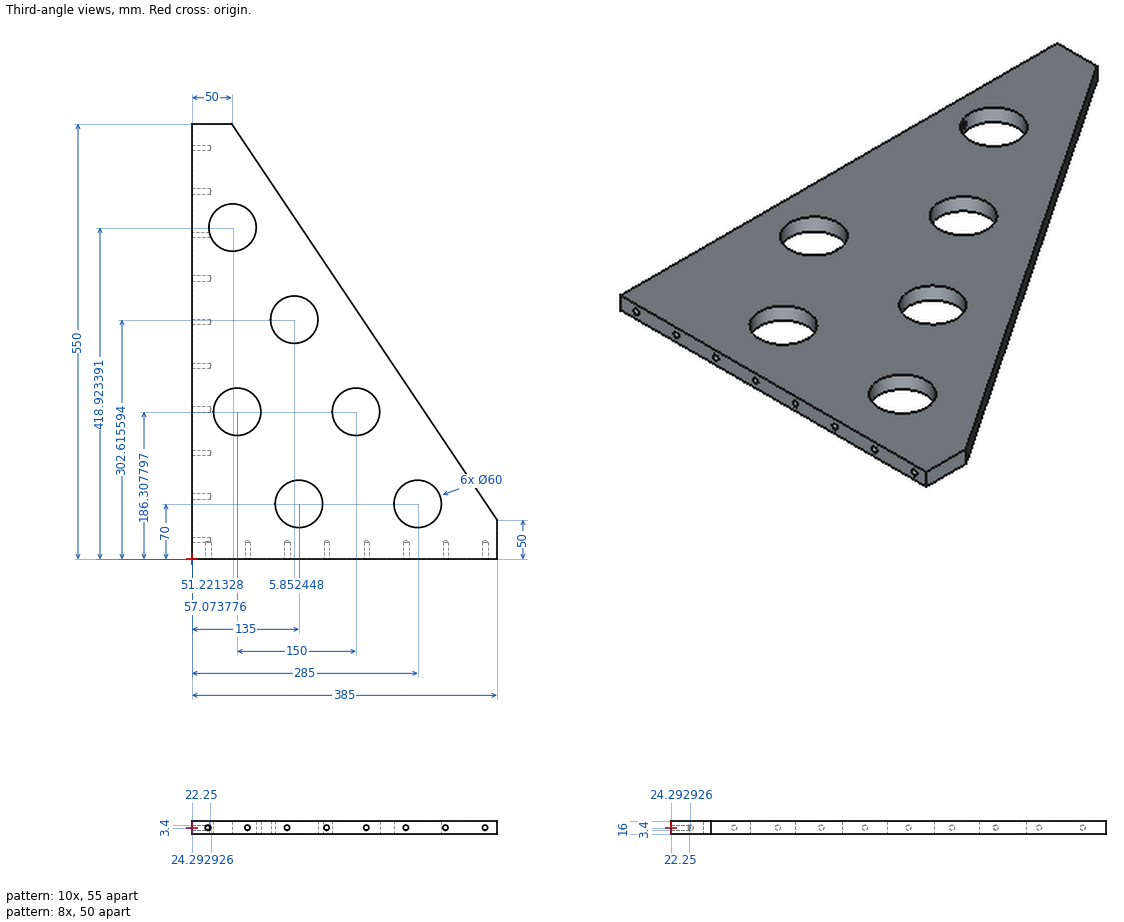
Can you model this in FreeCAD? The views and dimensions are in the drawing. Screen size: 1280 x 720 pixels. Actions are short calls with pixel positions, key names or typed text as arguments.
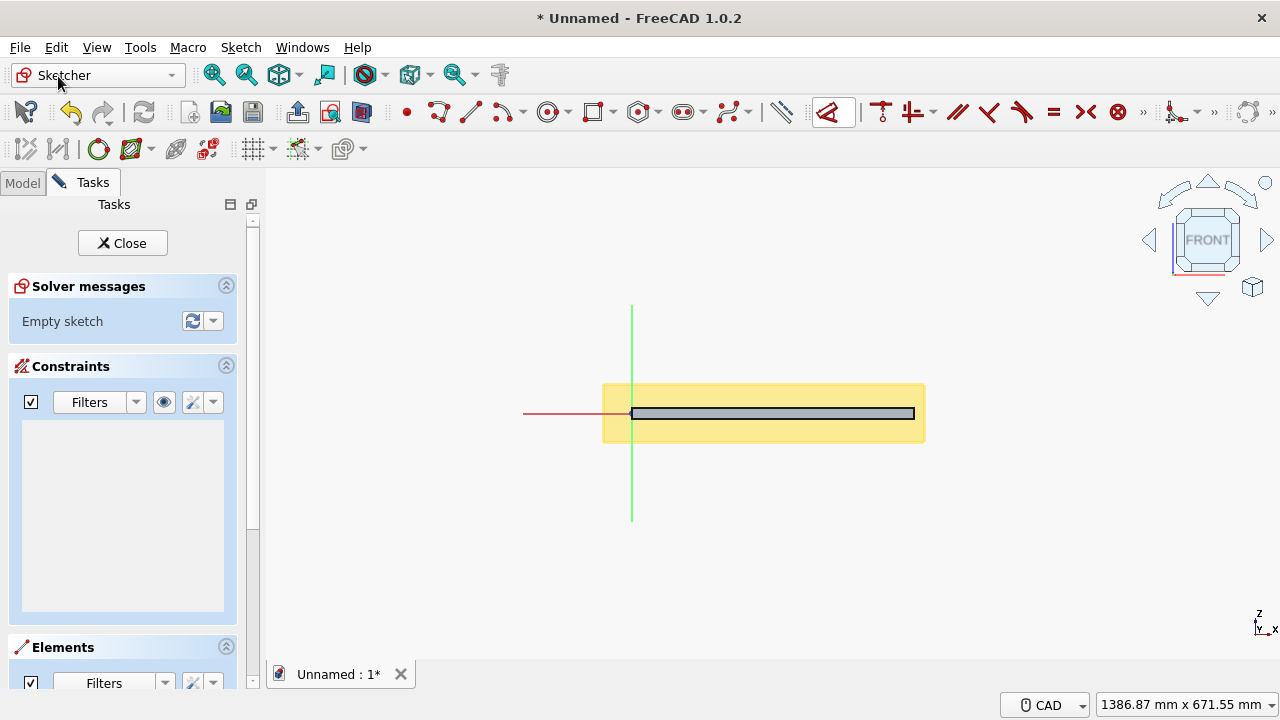
click(362, 112)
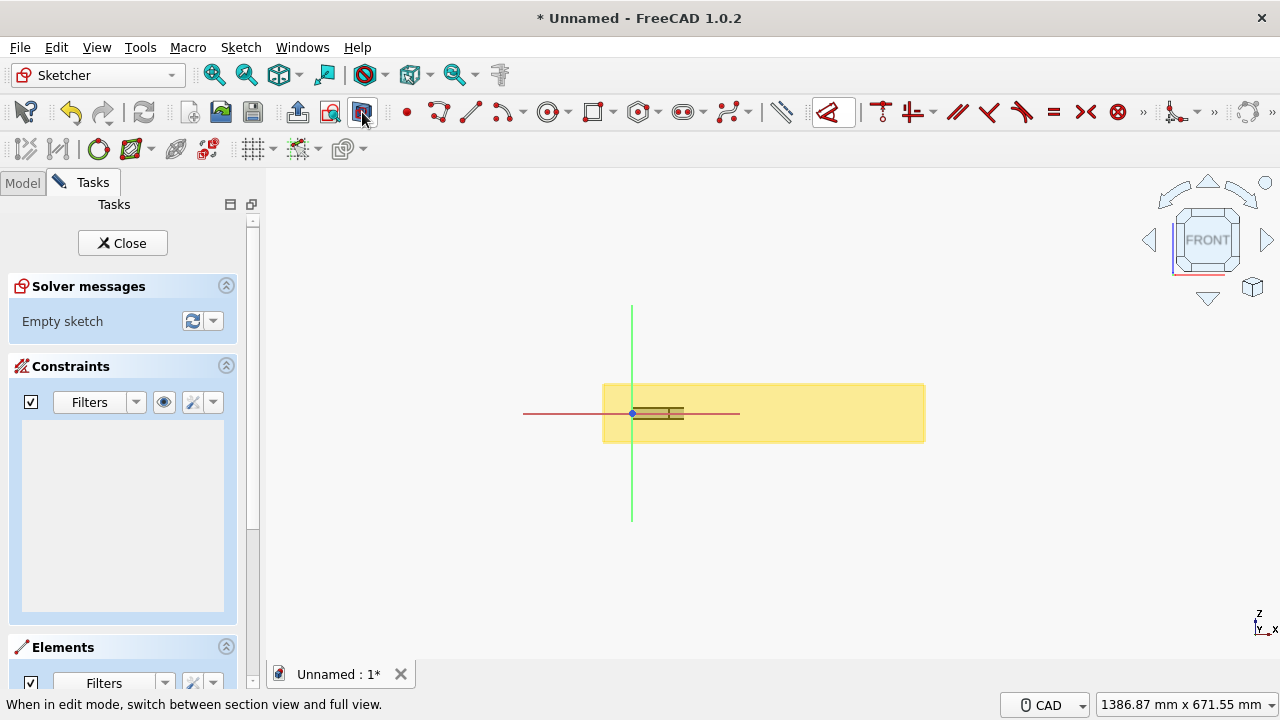
scroll(638, 412, up, 15)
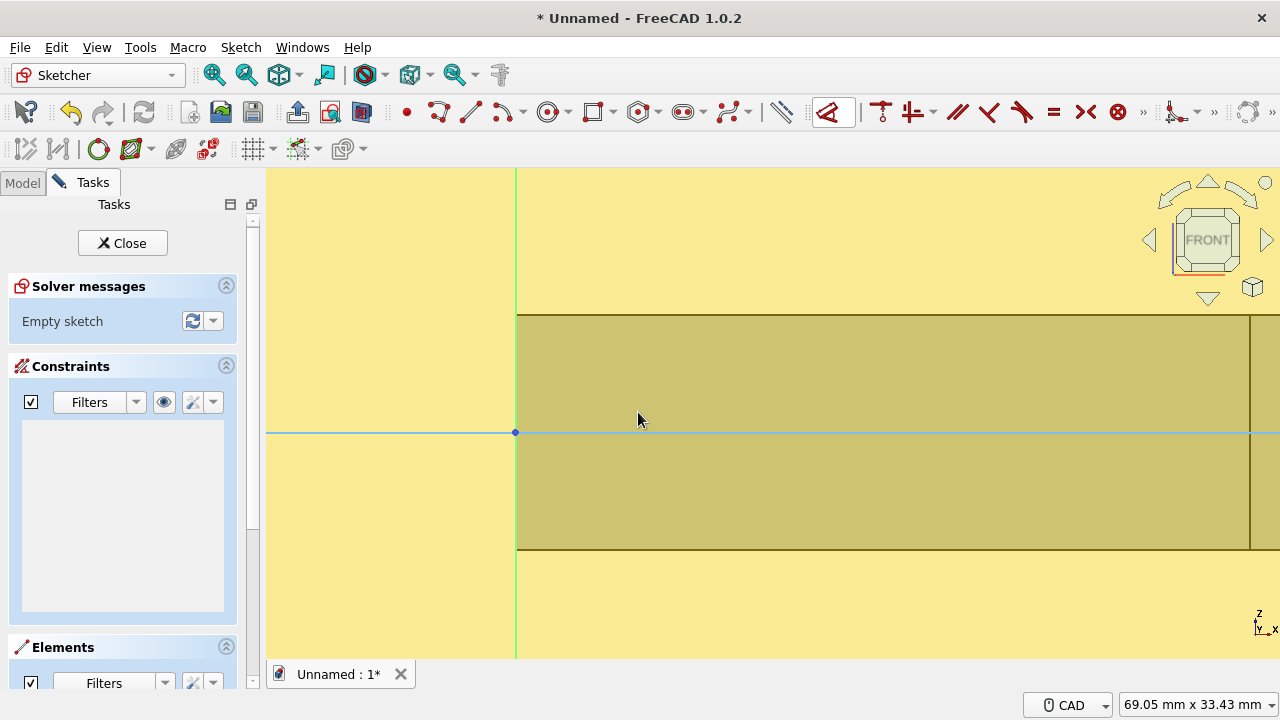
scroll(673, 396, up, 2)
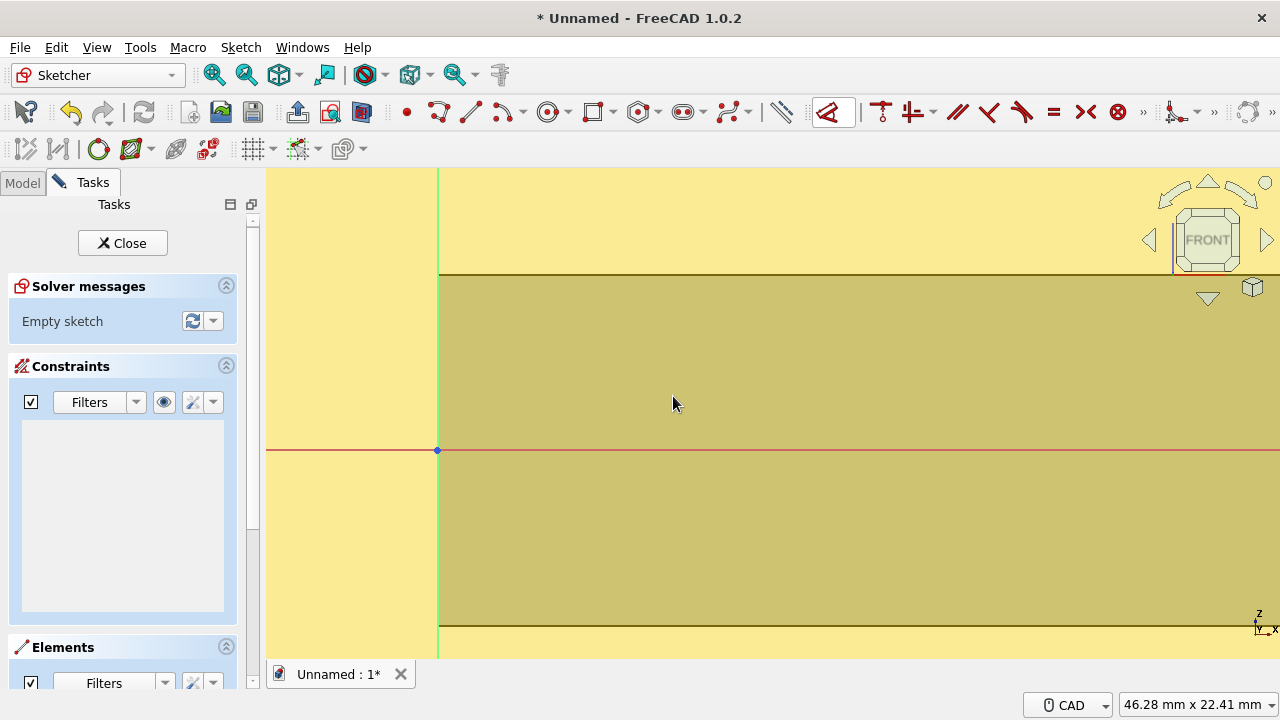
click(440, 112)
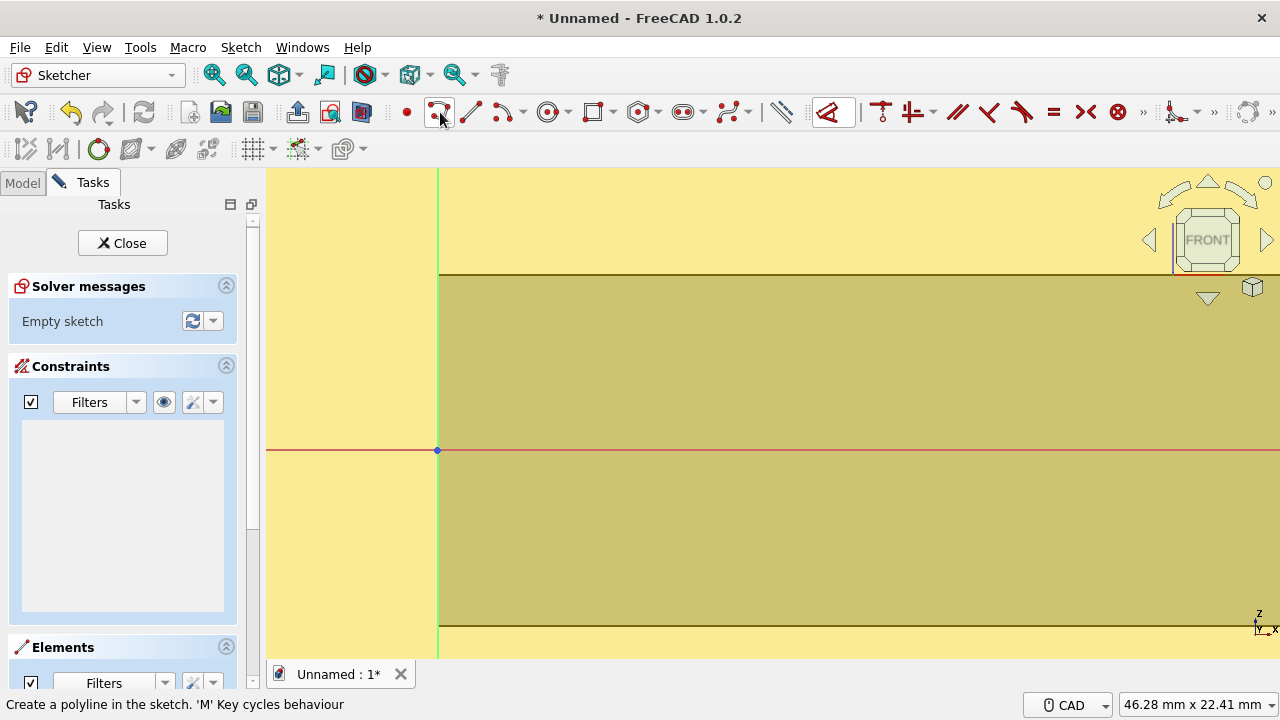
click(438, 450)
click(447, 376)
click(925, 376)
click(970, 441)
click(438, 450)
key(Escape)
key(Escape)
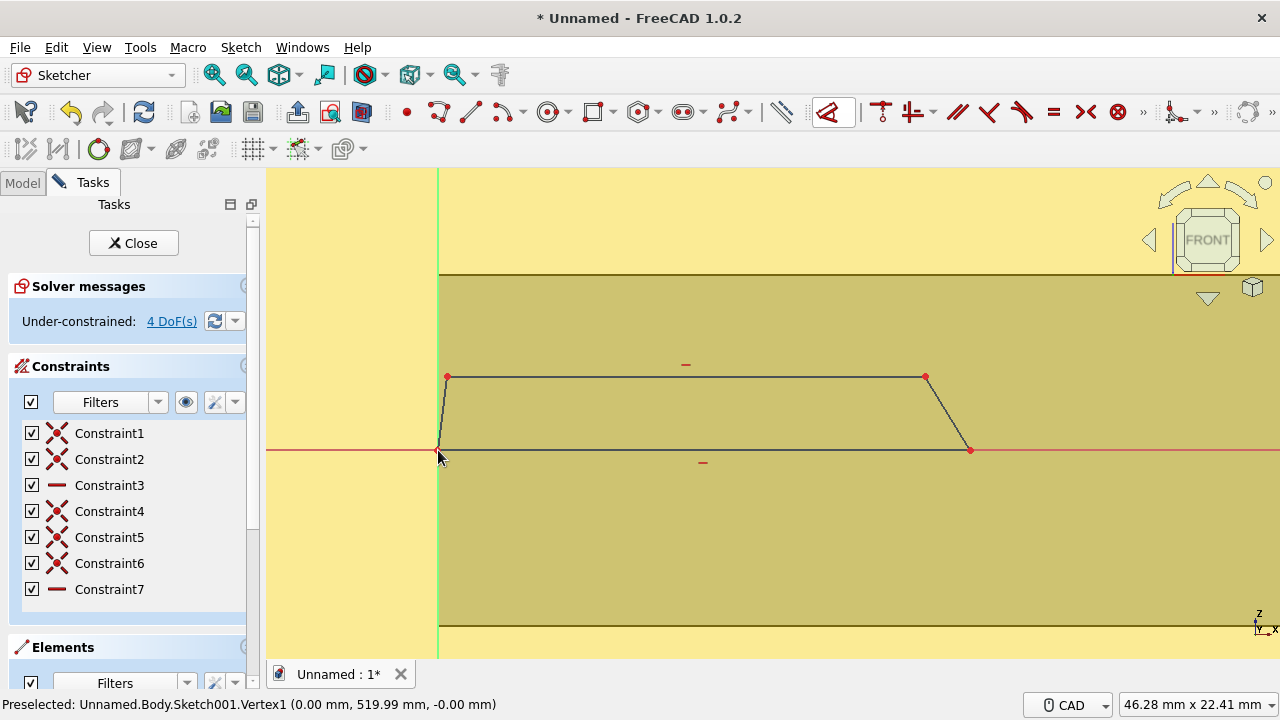
click(441, 428)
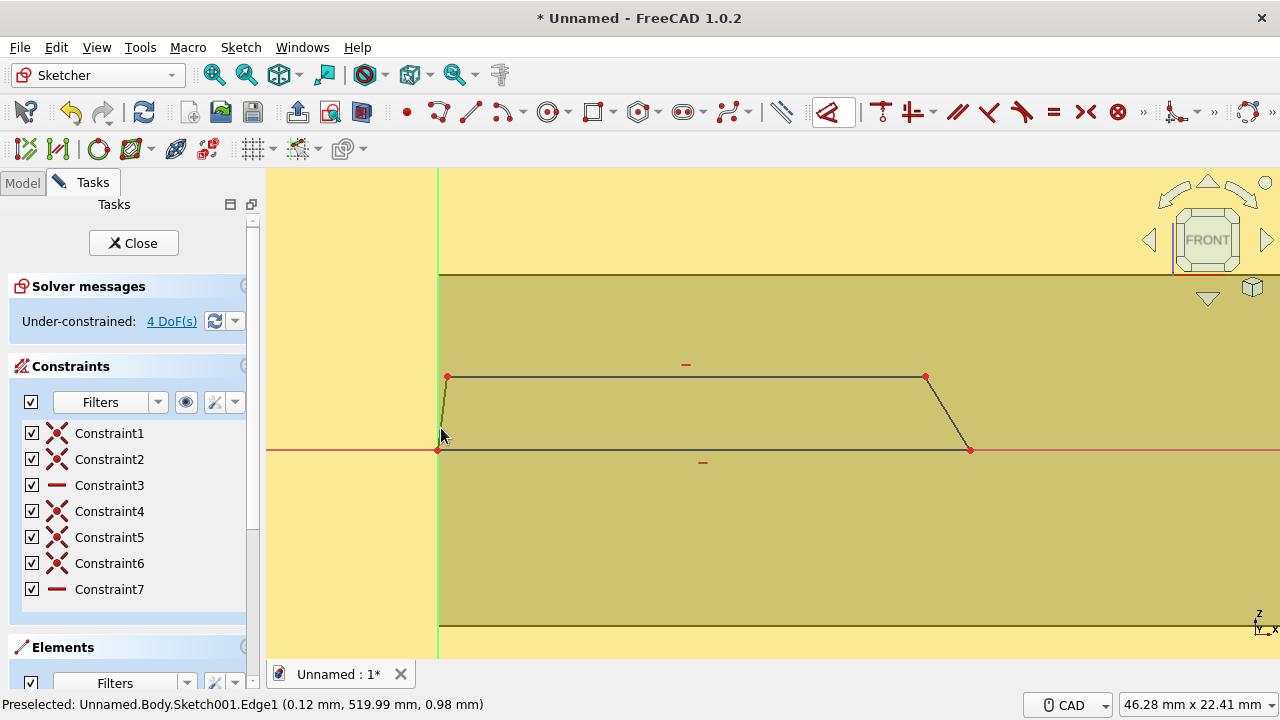
key(v)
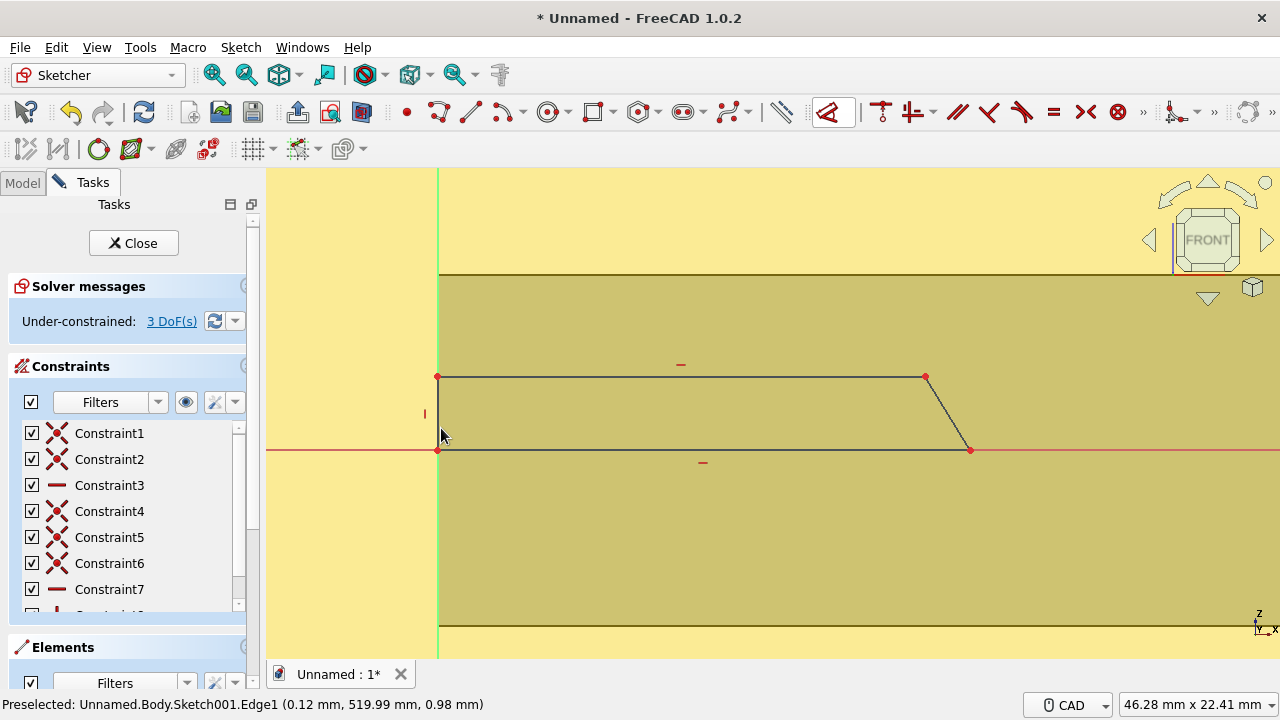
click(438, 428)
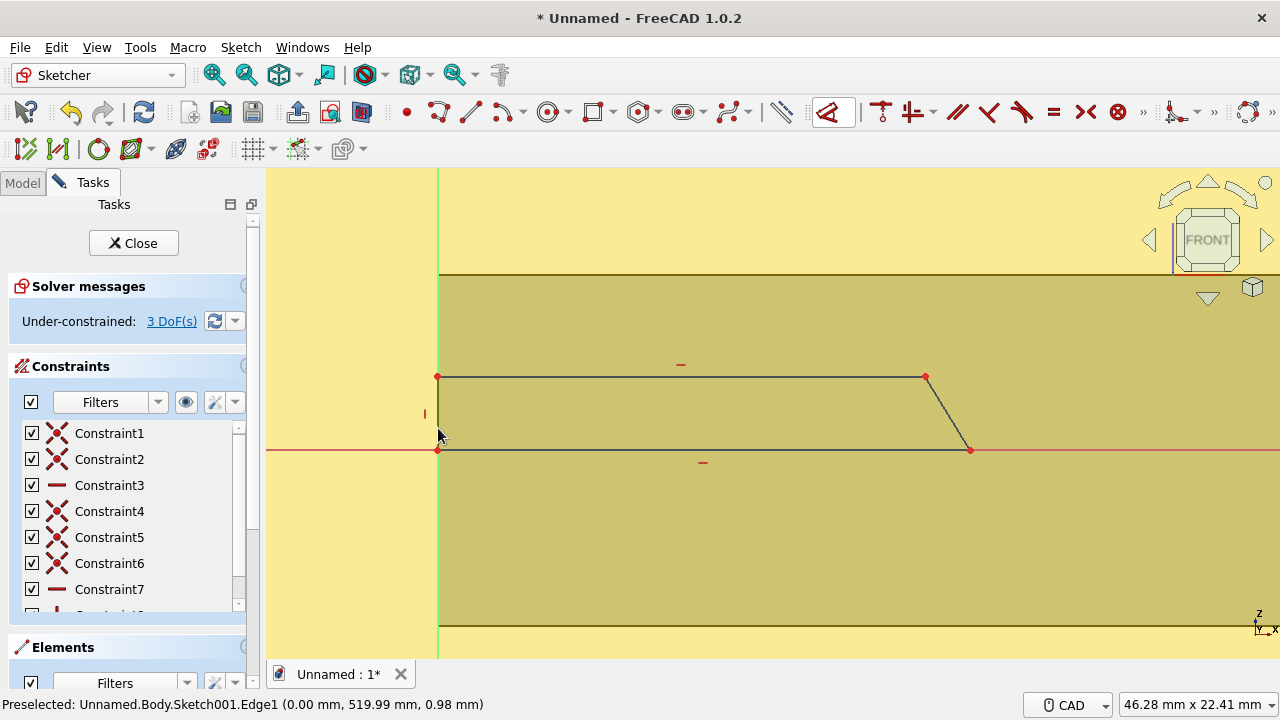
click(850, 112)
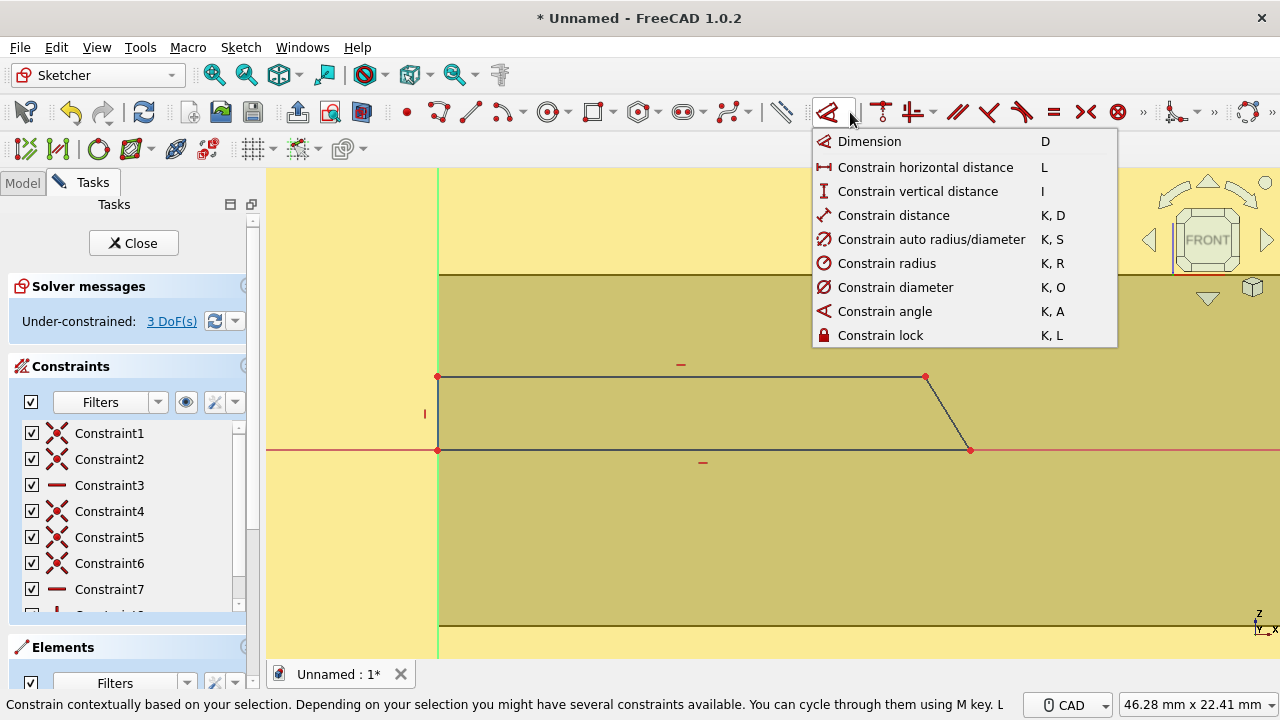
click(965, 191)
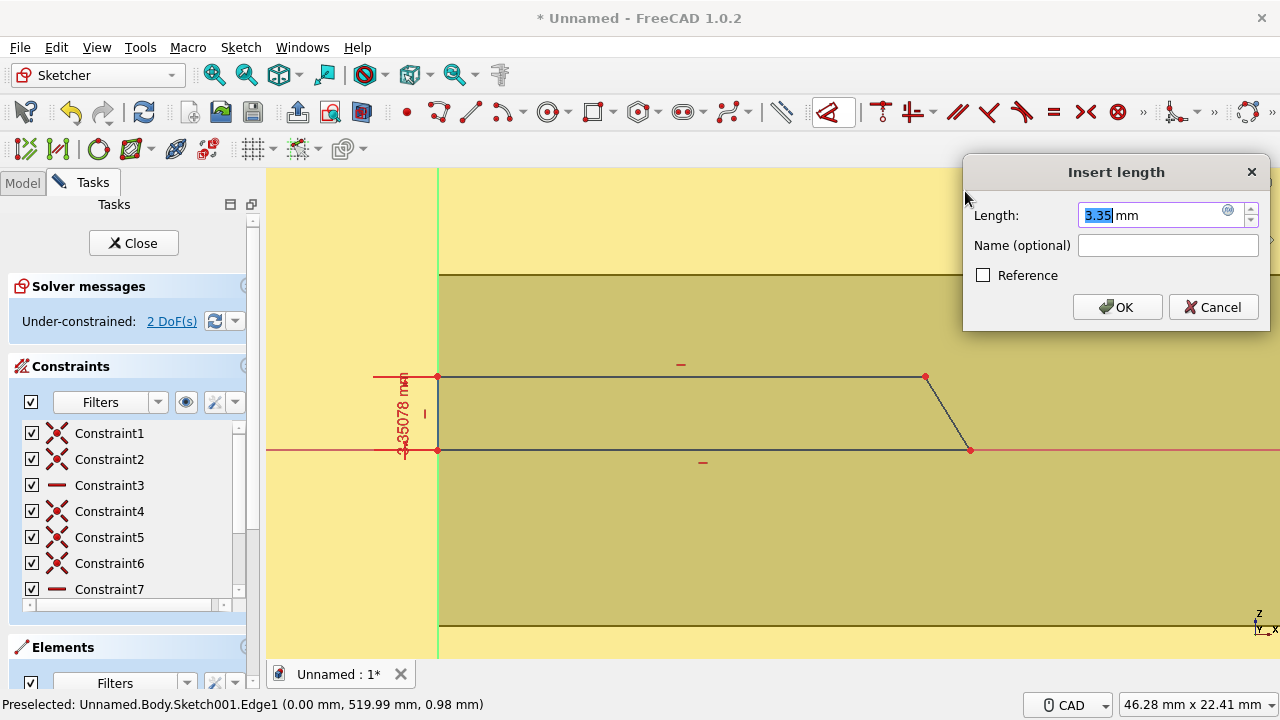
text(3.4)
key(Return)